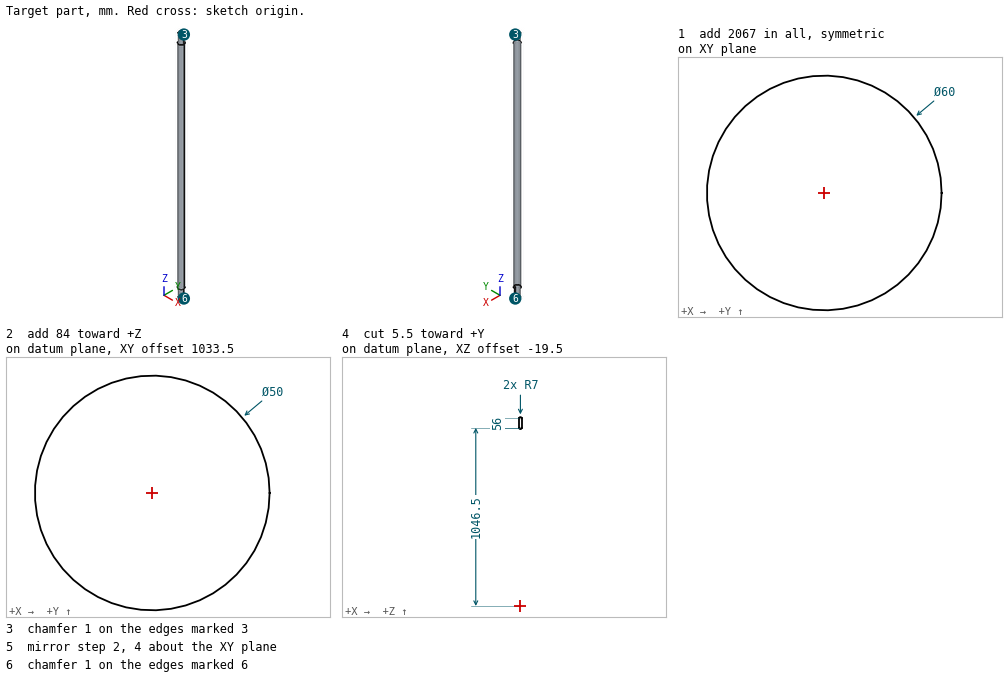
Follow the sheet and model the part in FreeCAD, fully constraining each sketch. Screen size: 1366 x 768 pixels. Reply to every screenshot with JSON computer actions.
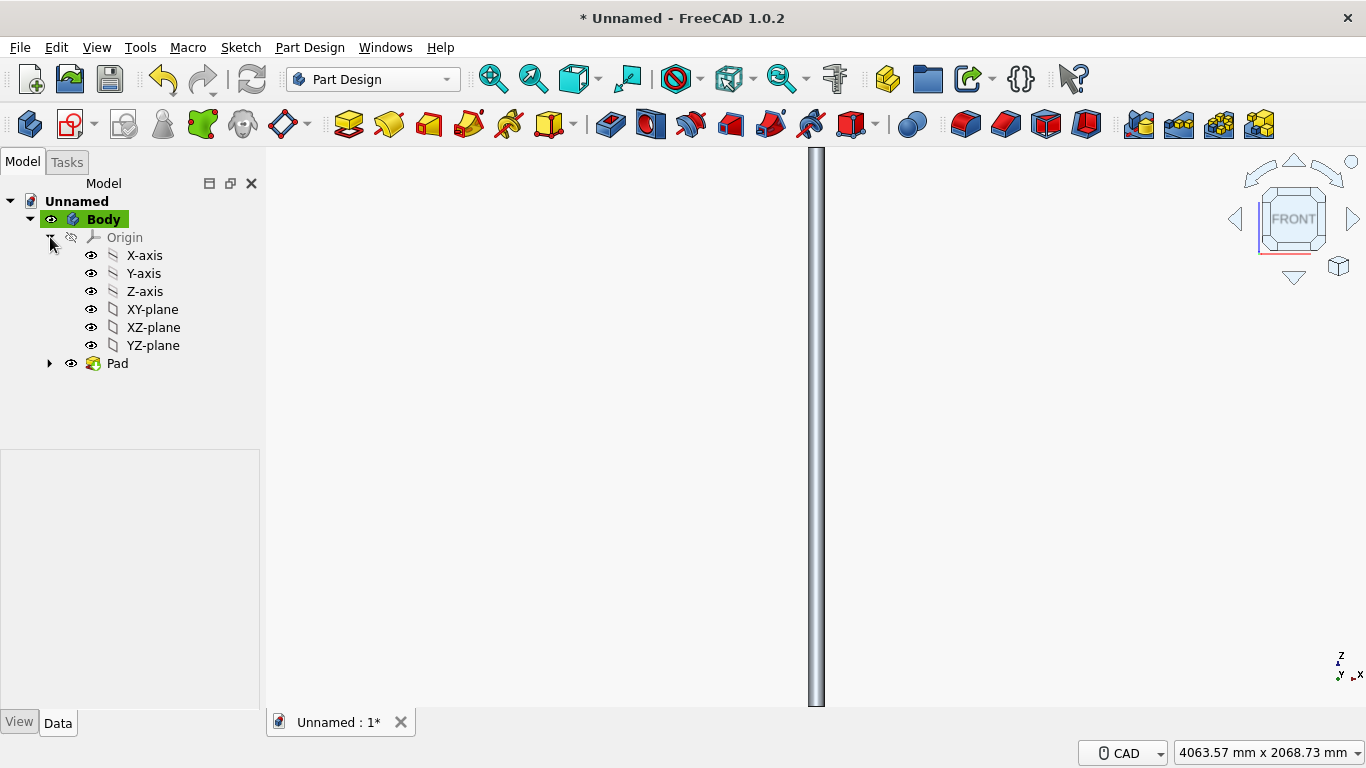
{"action": "left_click", "coordinate": [136, 309]}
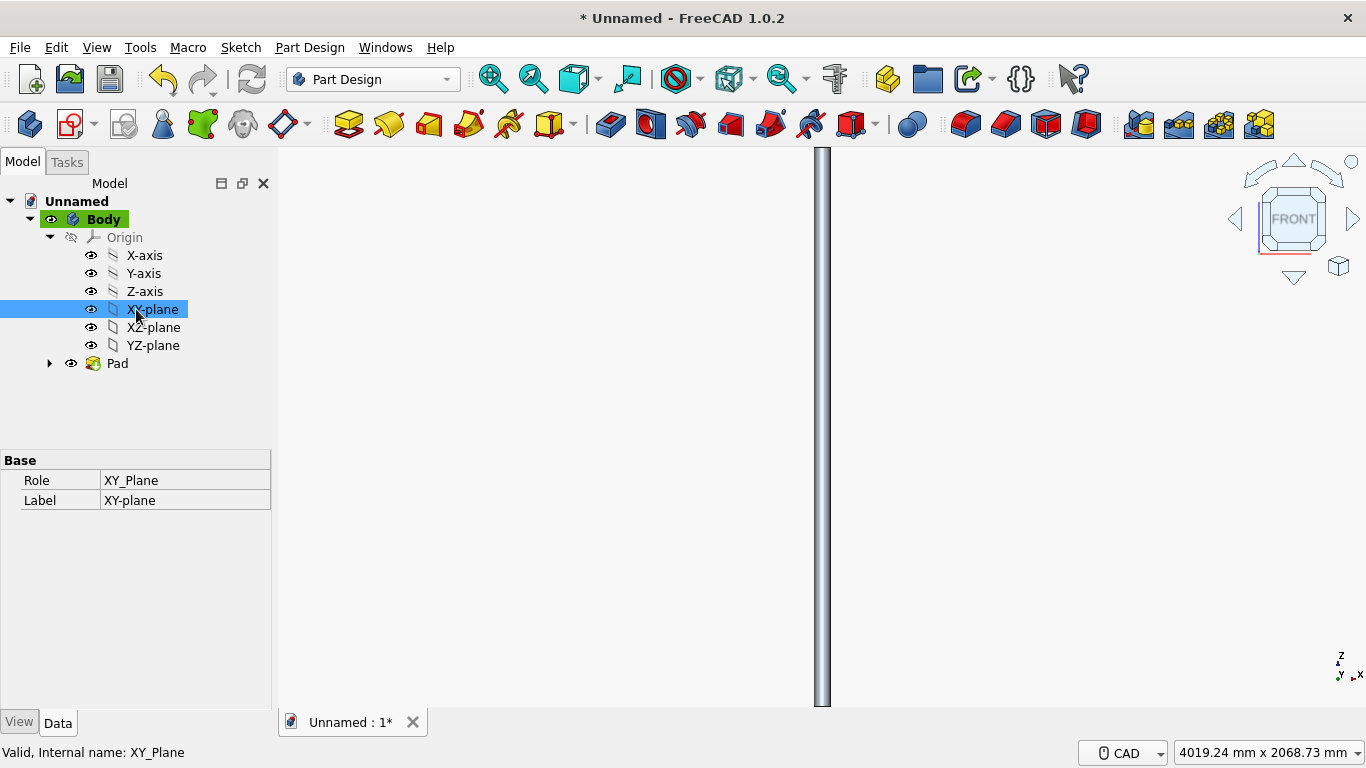
{"action": "left_click", "coordinate": [284, 124]}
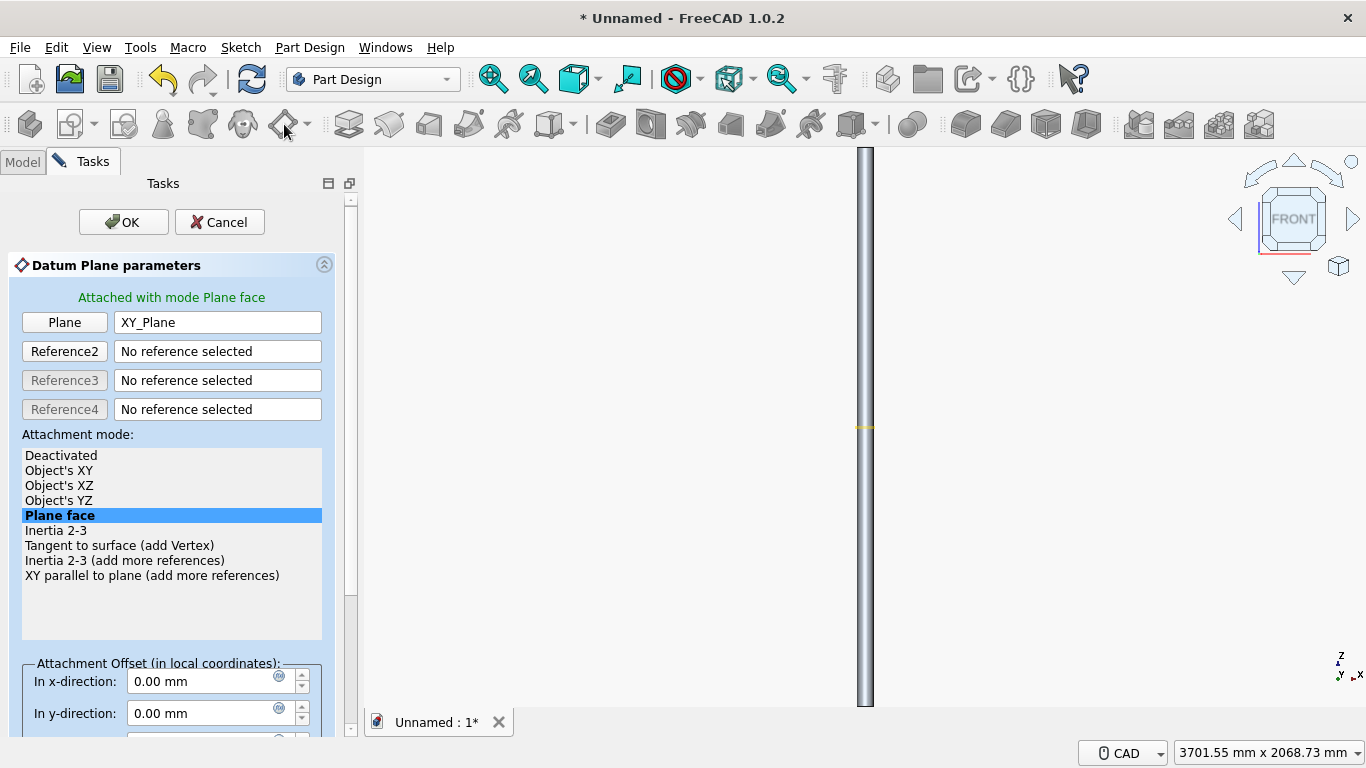
{"action": "scroll", "coordinate": [351, 464], "scroll_direction": "down", "scroll_amount": 2}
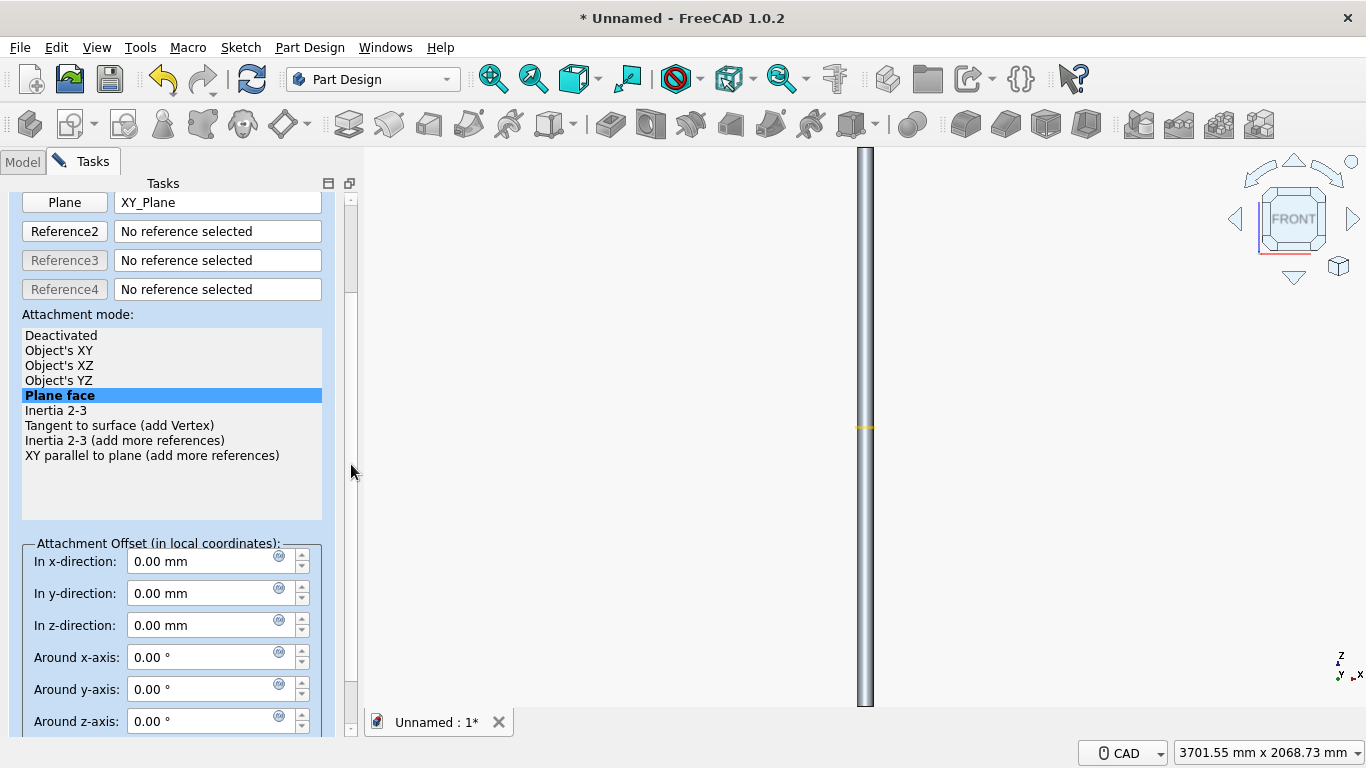
{"action": "triple_click", "coordinate": [210, 625]}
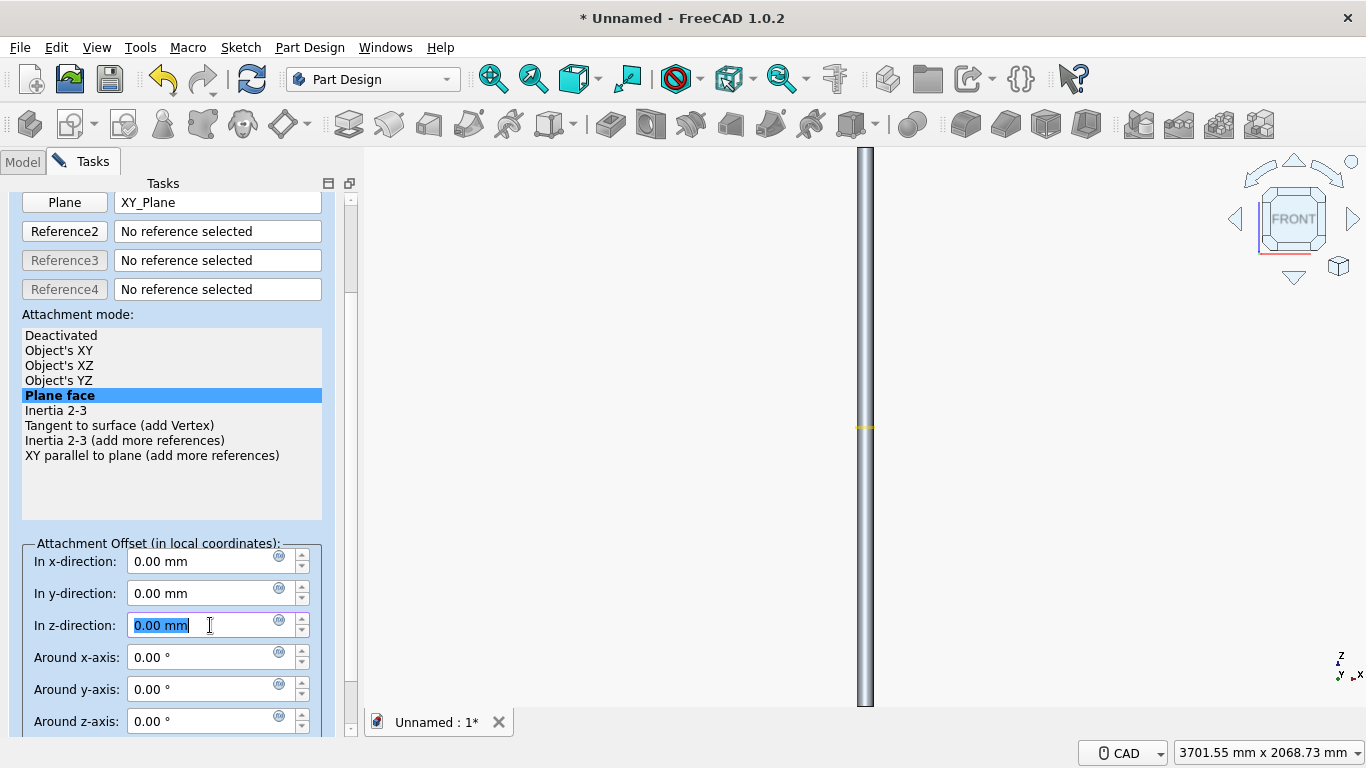
{"action": "type", "text": "1033.5"}
{"action": "key", "text": "Tab"}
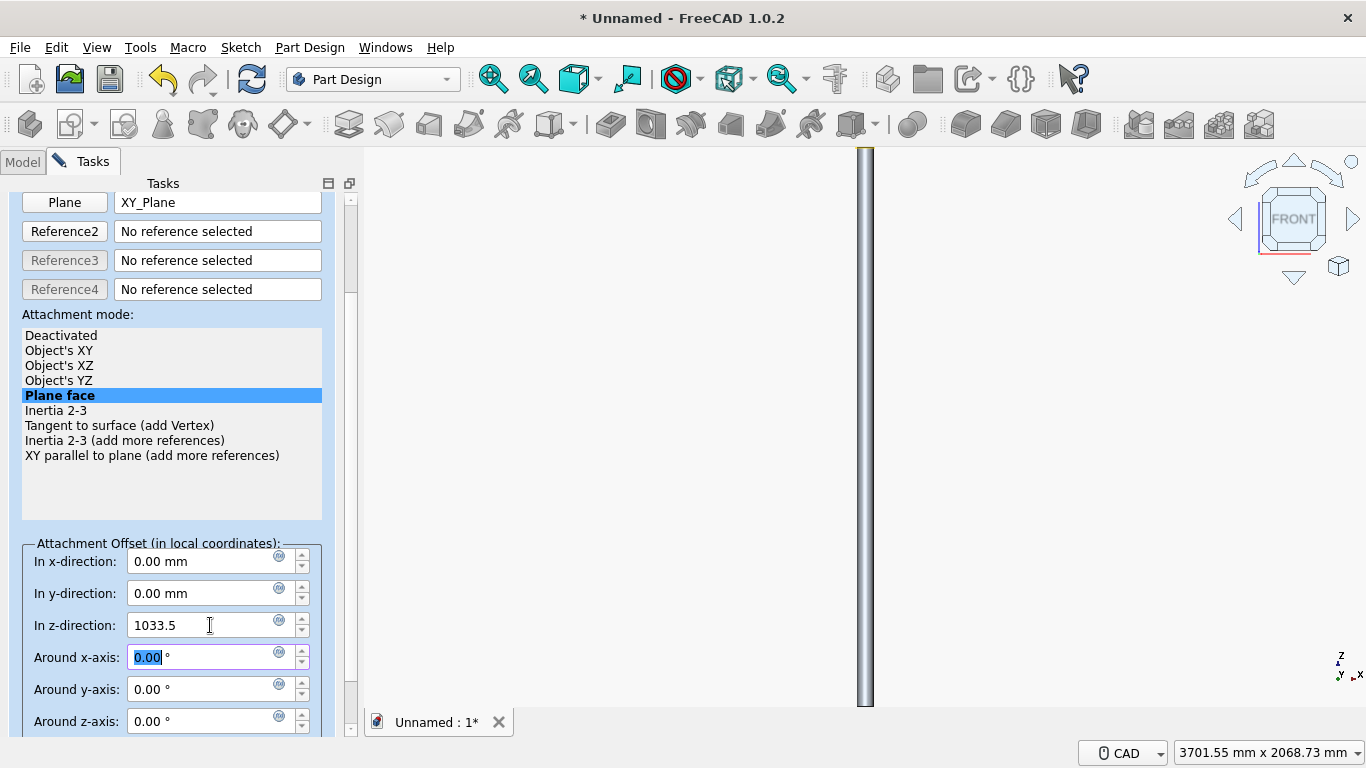
{"action": "scroll", "coordinate": [351, 464], "scroll_direction": "up", "scroll_amount": 3}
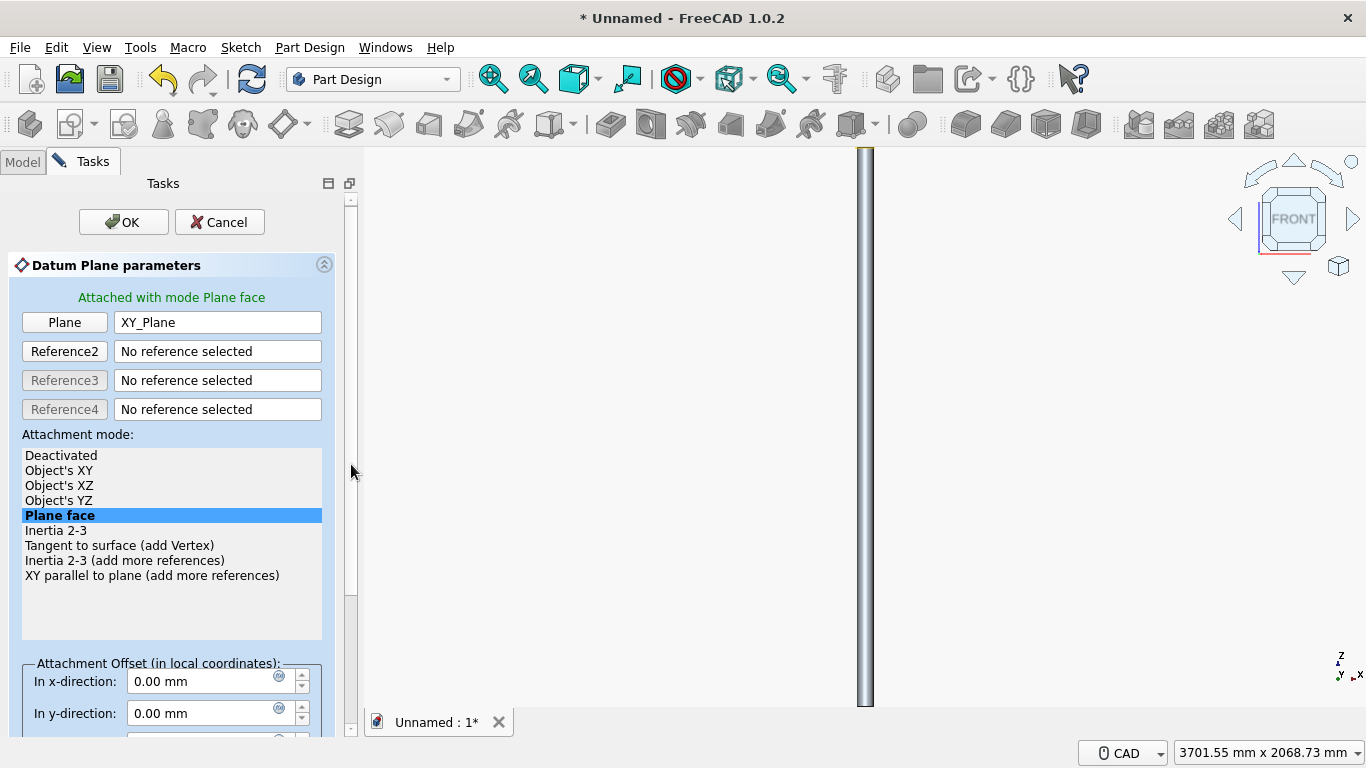
{"action": "left_click", "coordinate": [124, 222]}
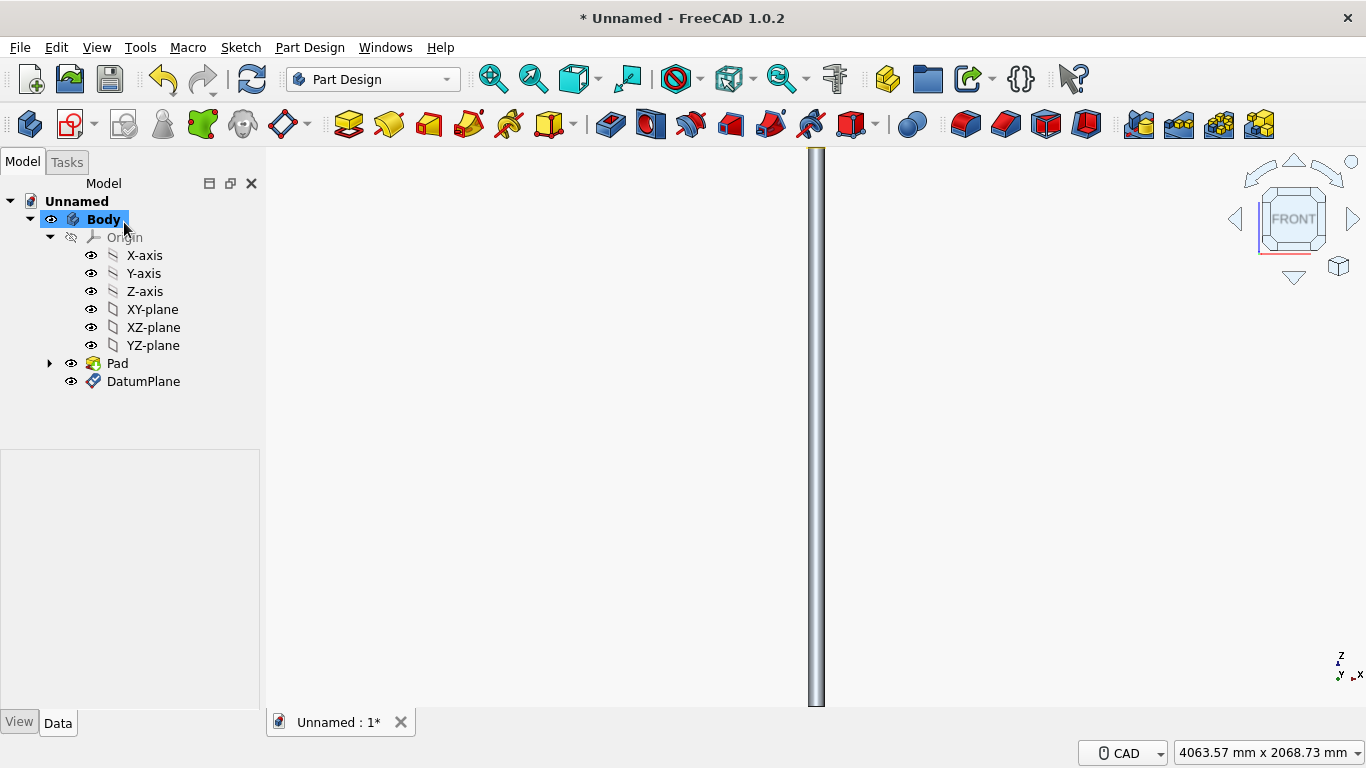
{"action": "left_click", "coordinate": [116, 381]}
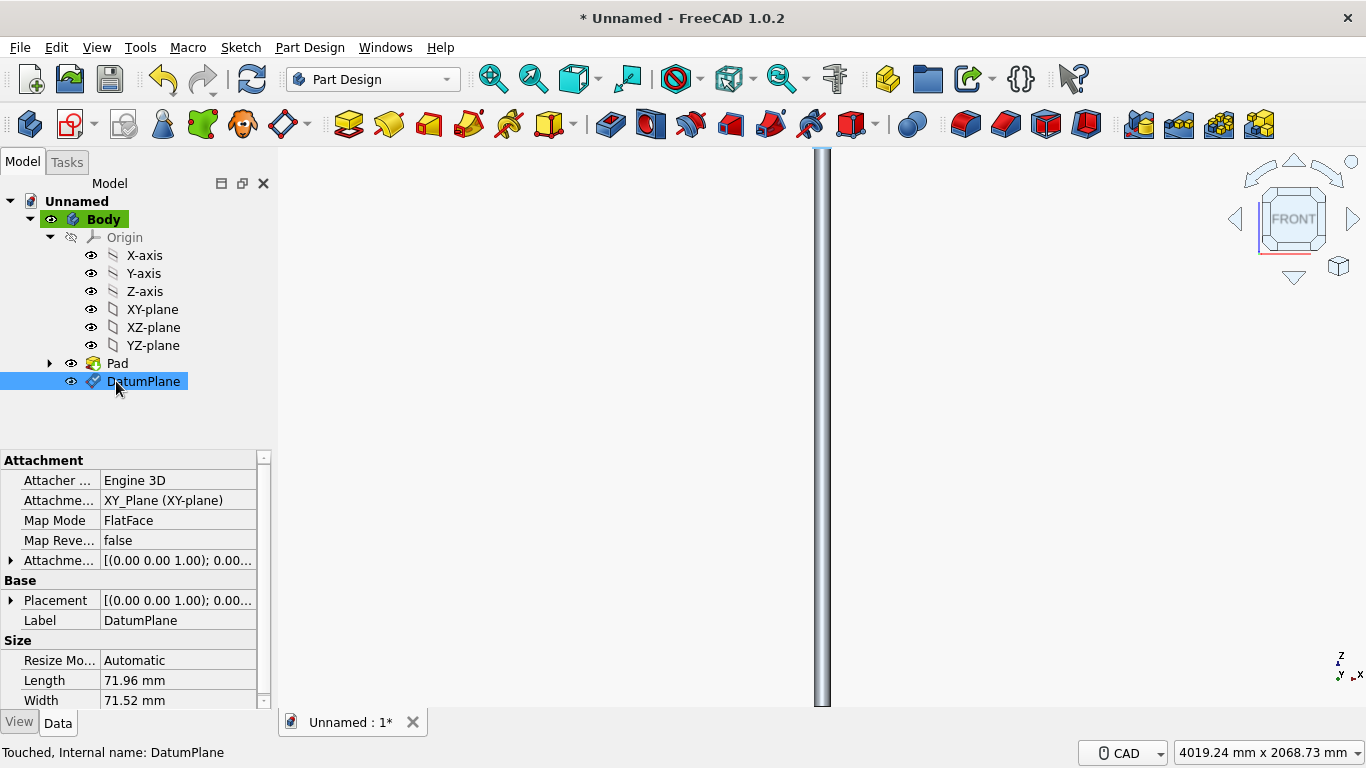
{"action": "left_click", "coordinate": [70, 124]}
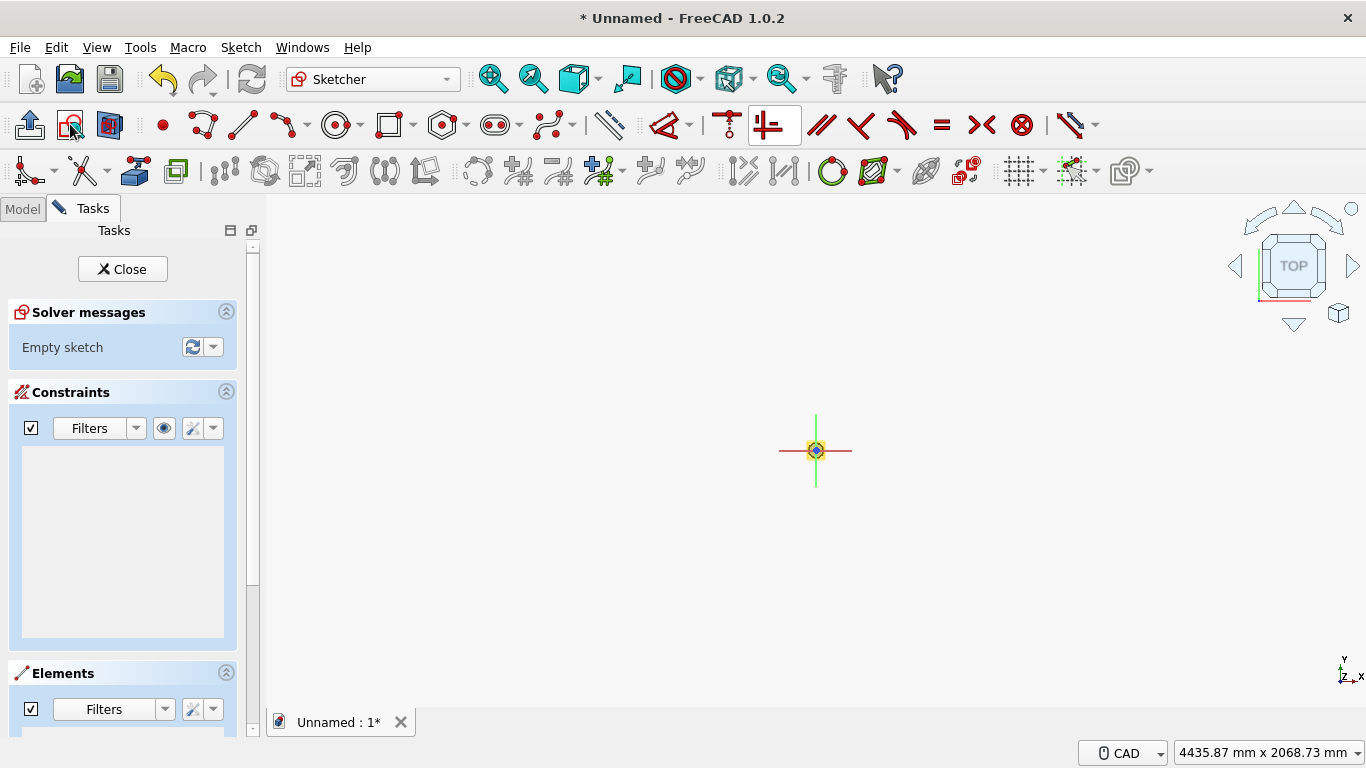
{"action": "scroll", "coordinate": [820, 451], "scroll_direction": "up", "scroll_amount": 15}